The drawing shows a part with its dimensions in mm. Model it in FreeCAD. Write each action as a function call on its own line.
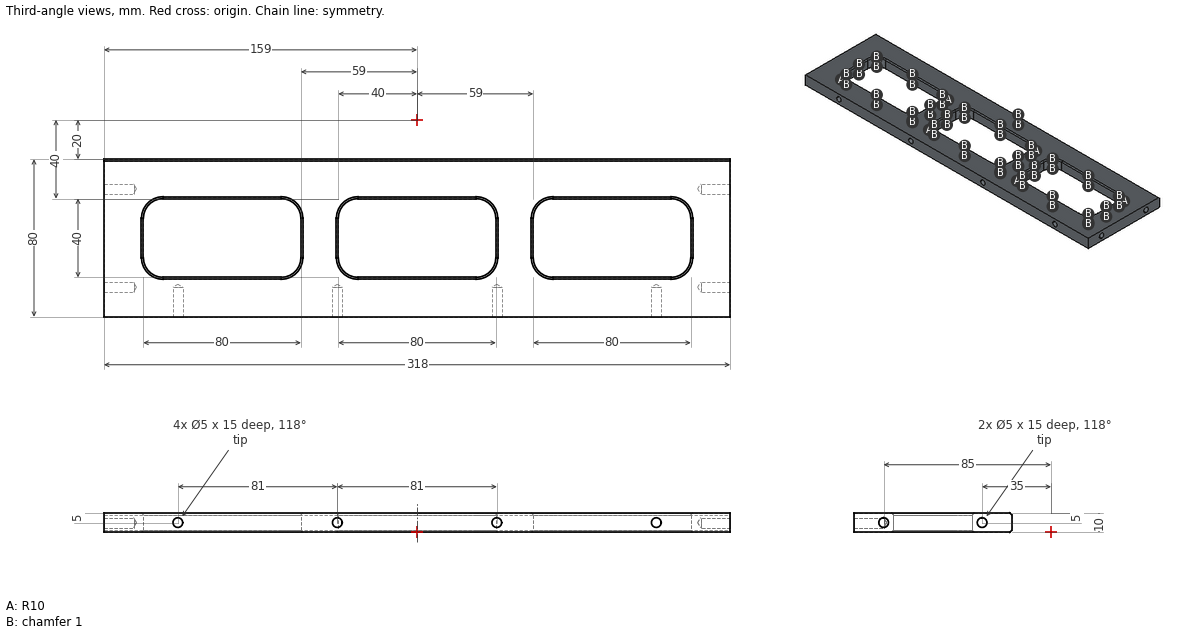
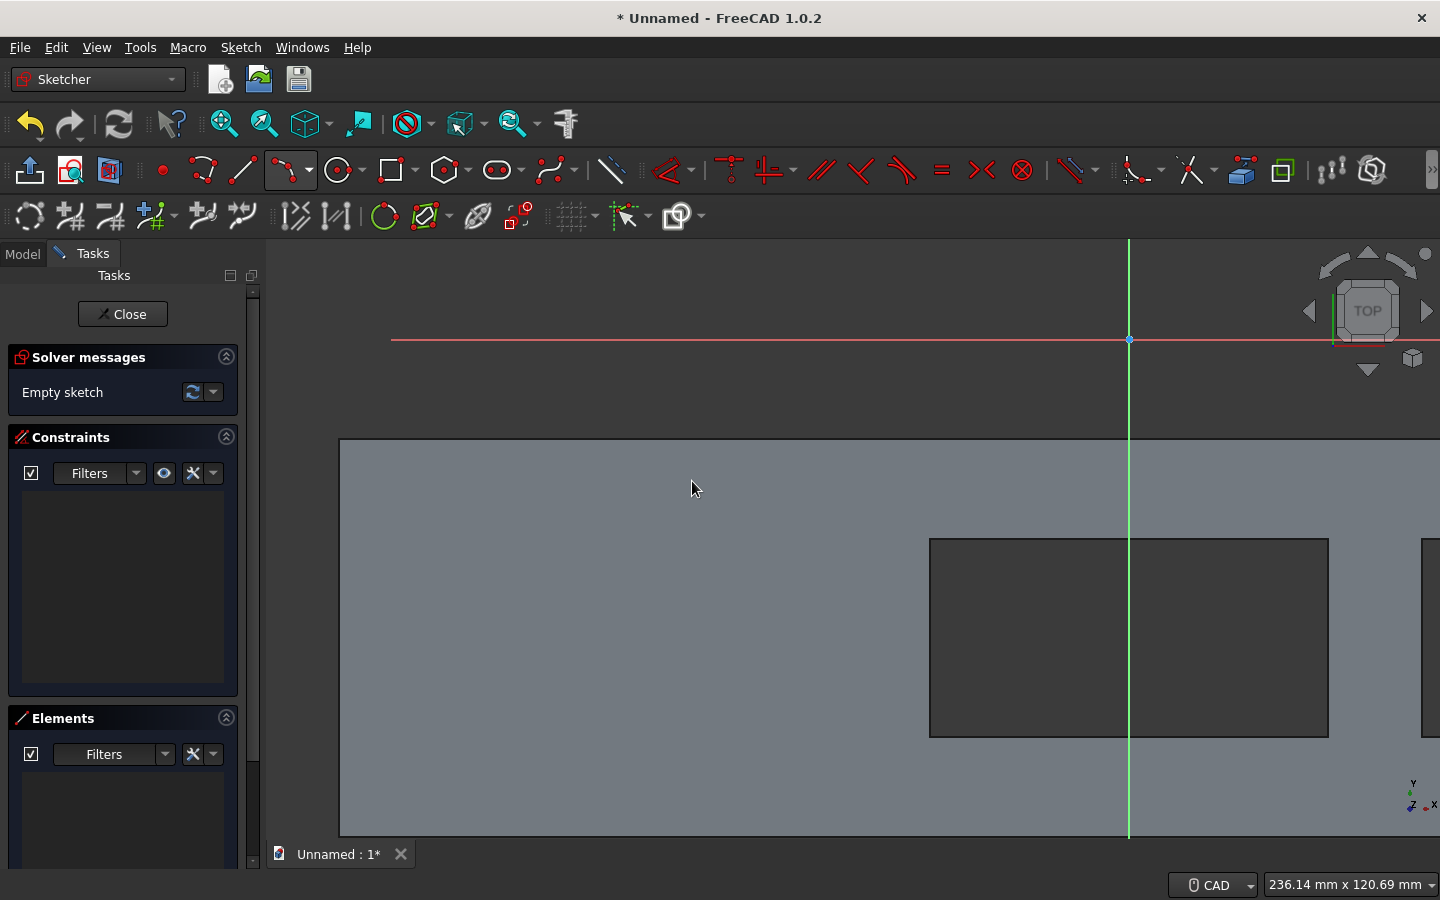
click(392, 170)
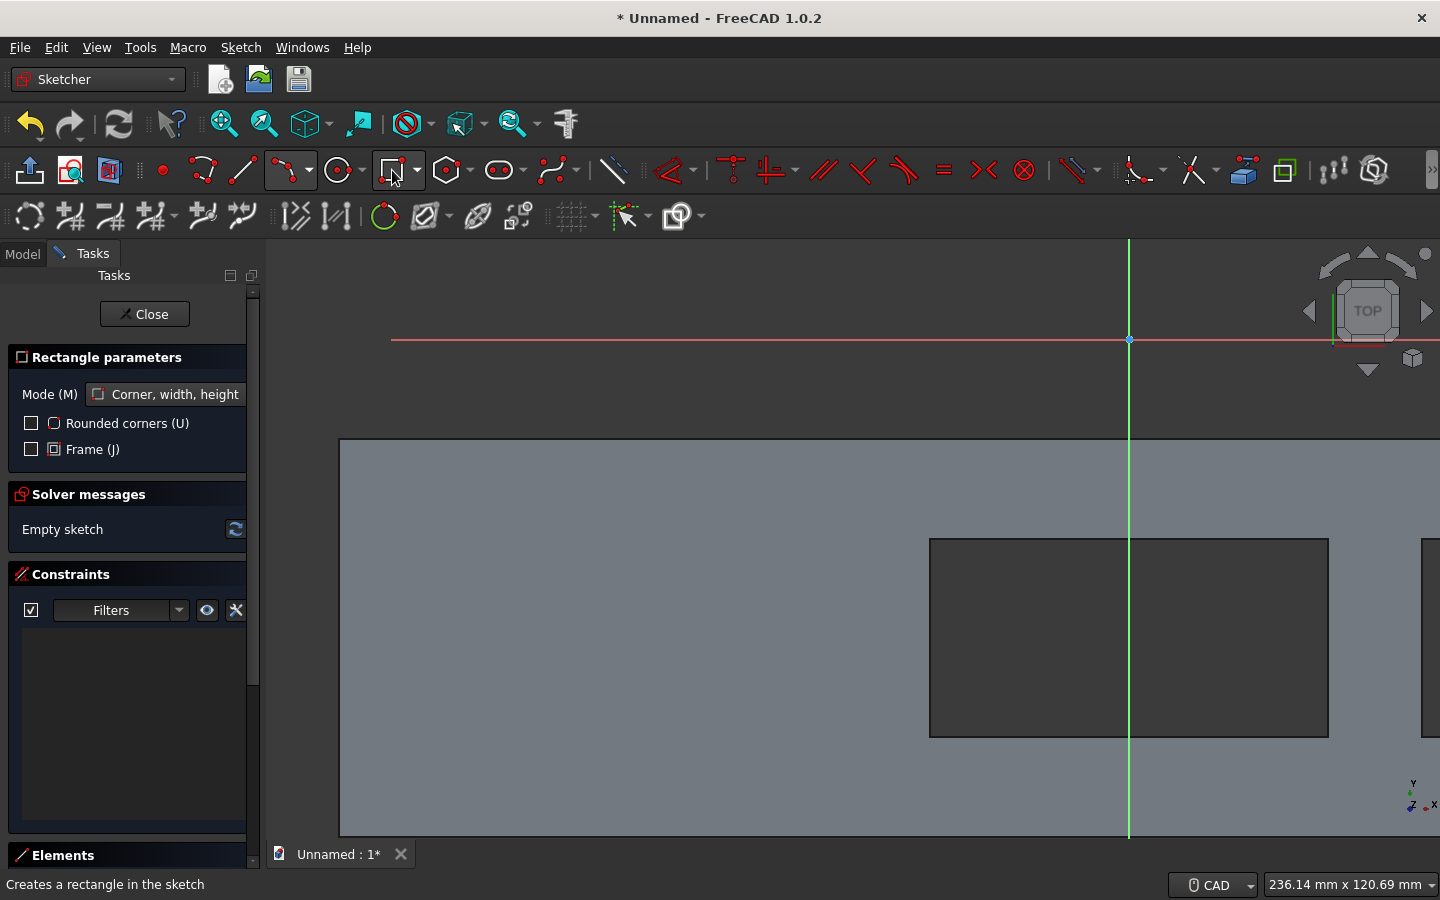
click(438, 539)
click(836, 737)
key(Escape)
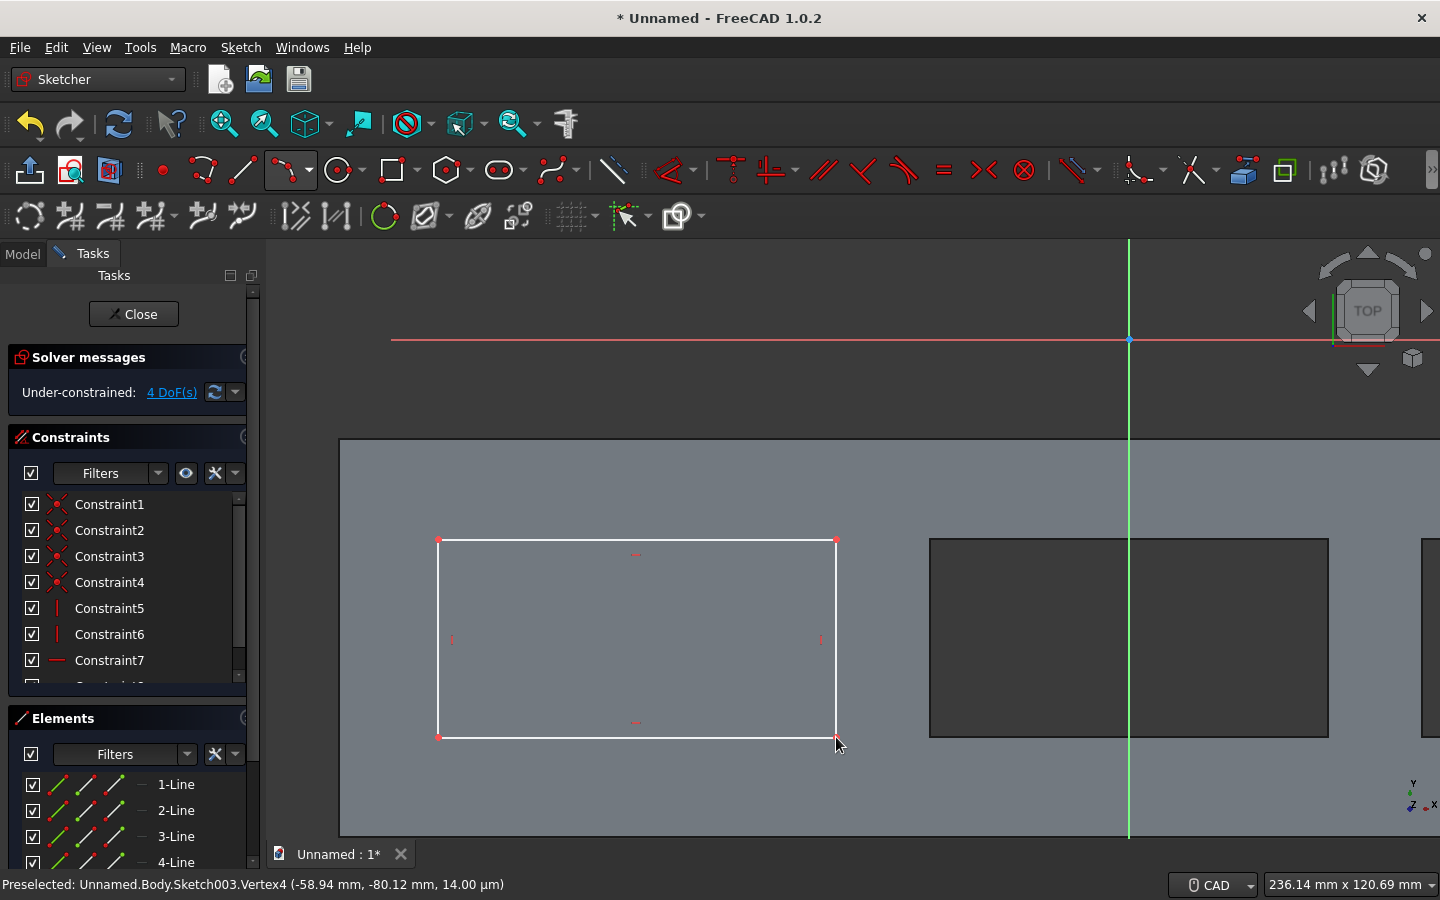
click(668, 170)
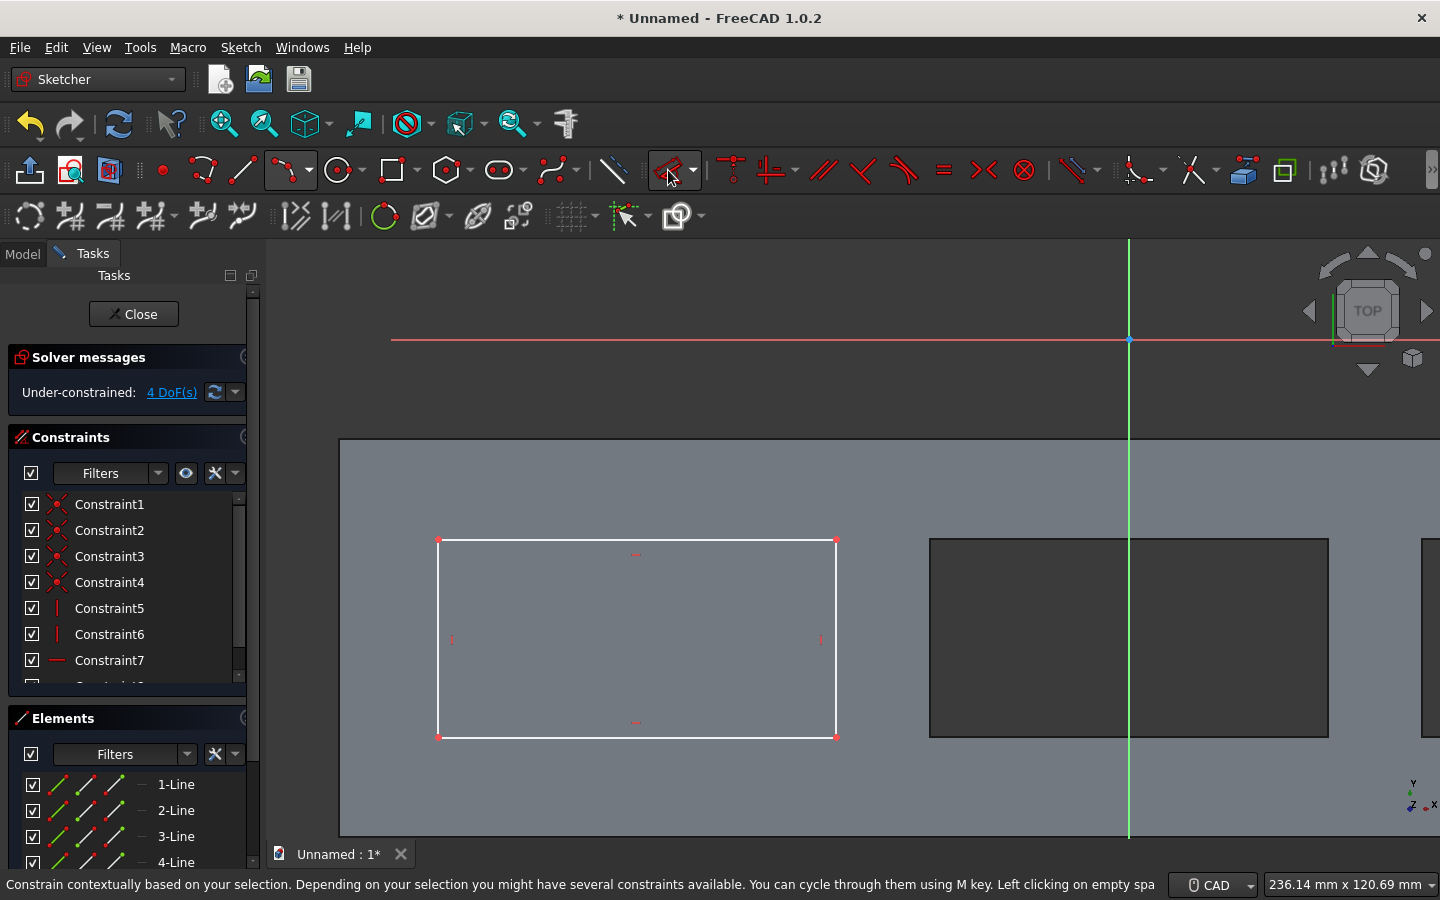
click(438, 599)
click(404, 639)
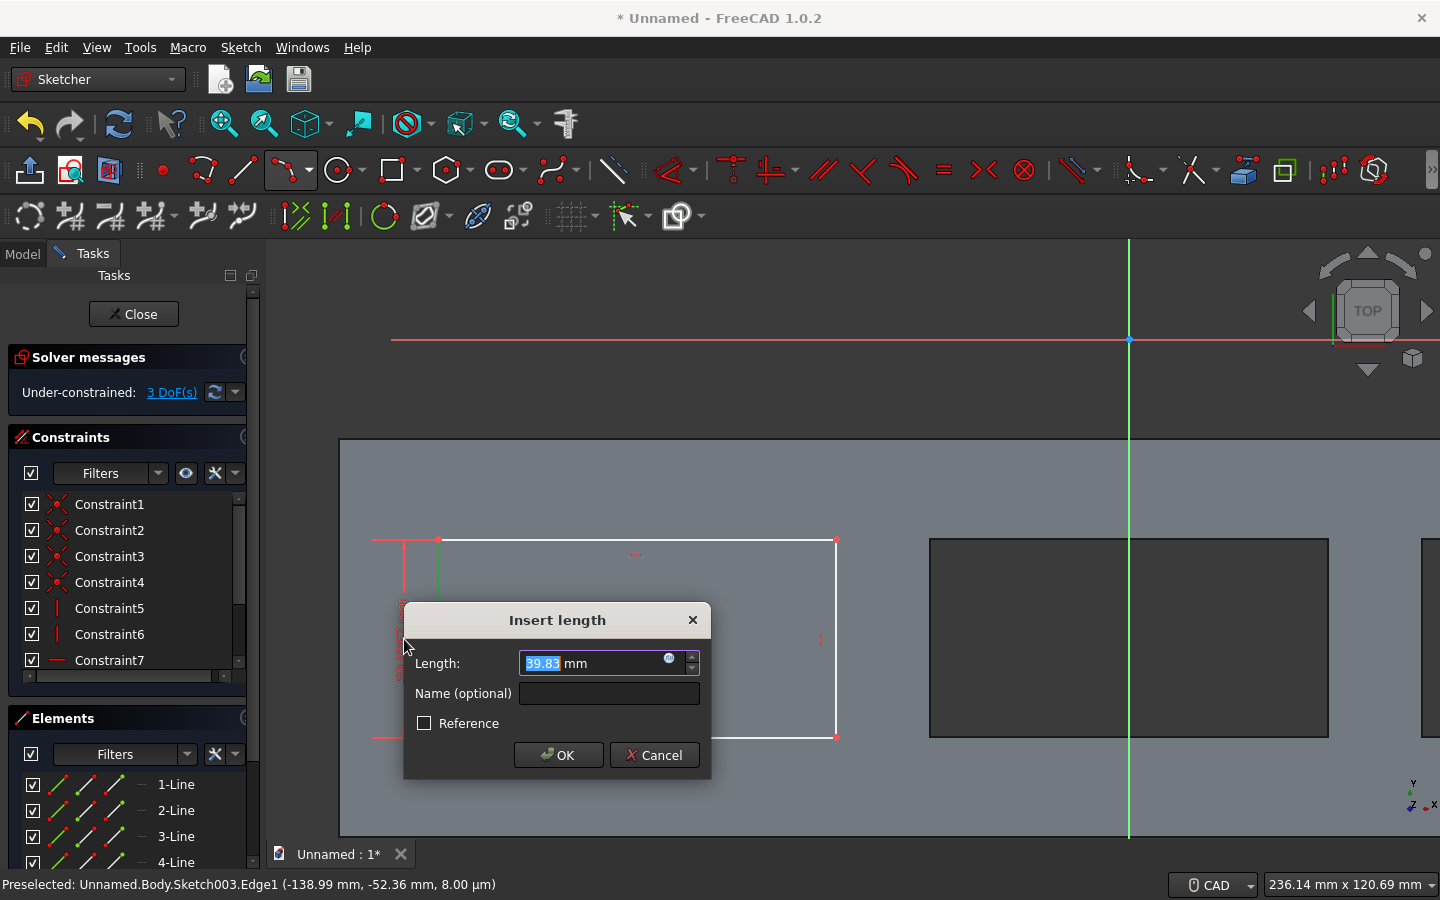
text(40)
key(Return)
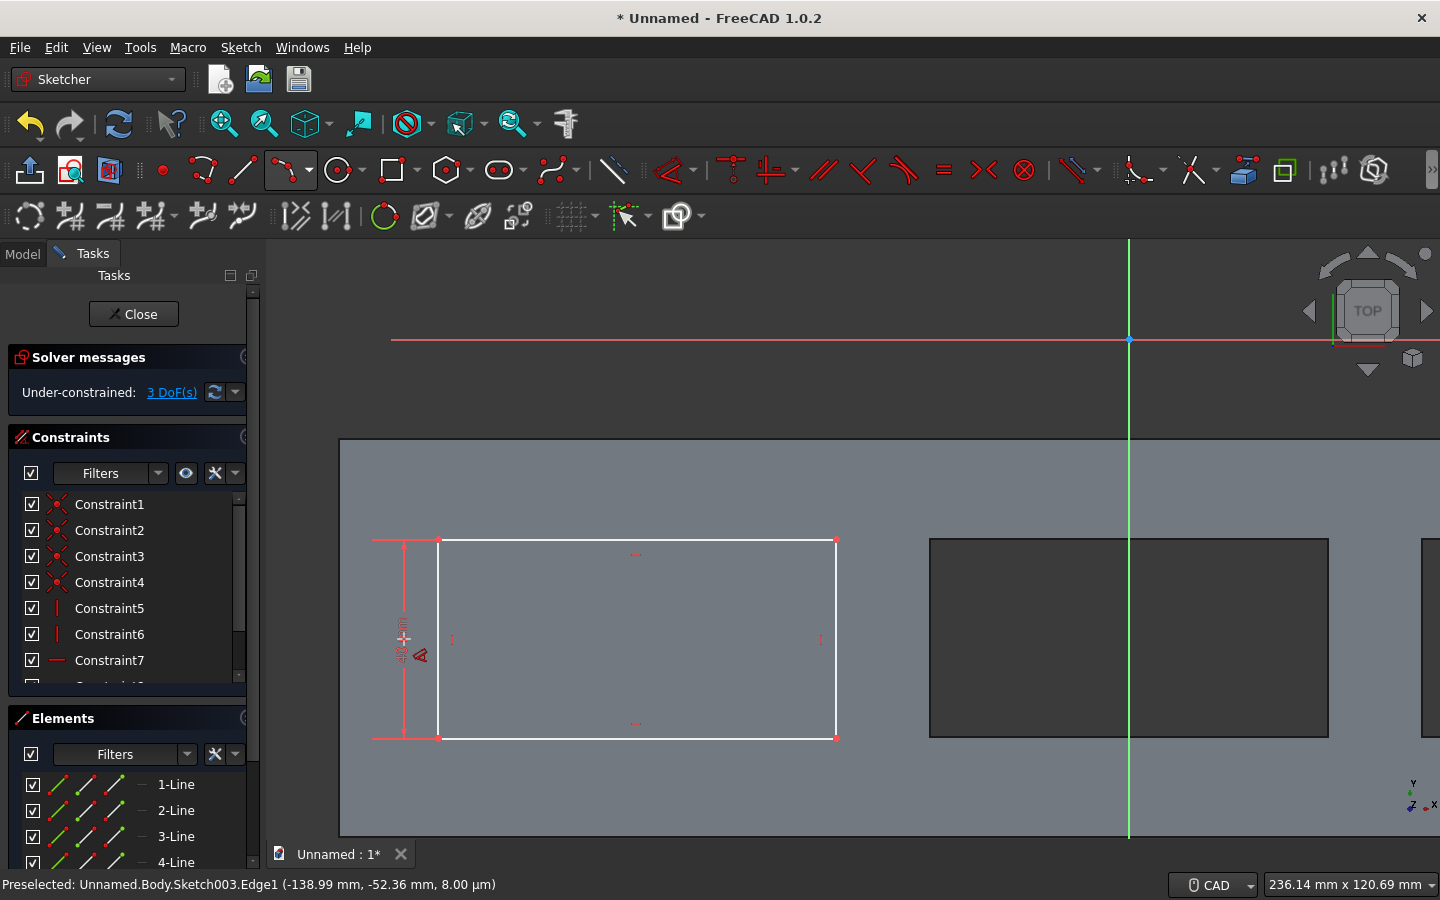
click(557, 739)
click(637, 773)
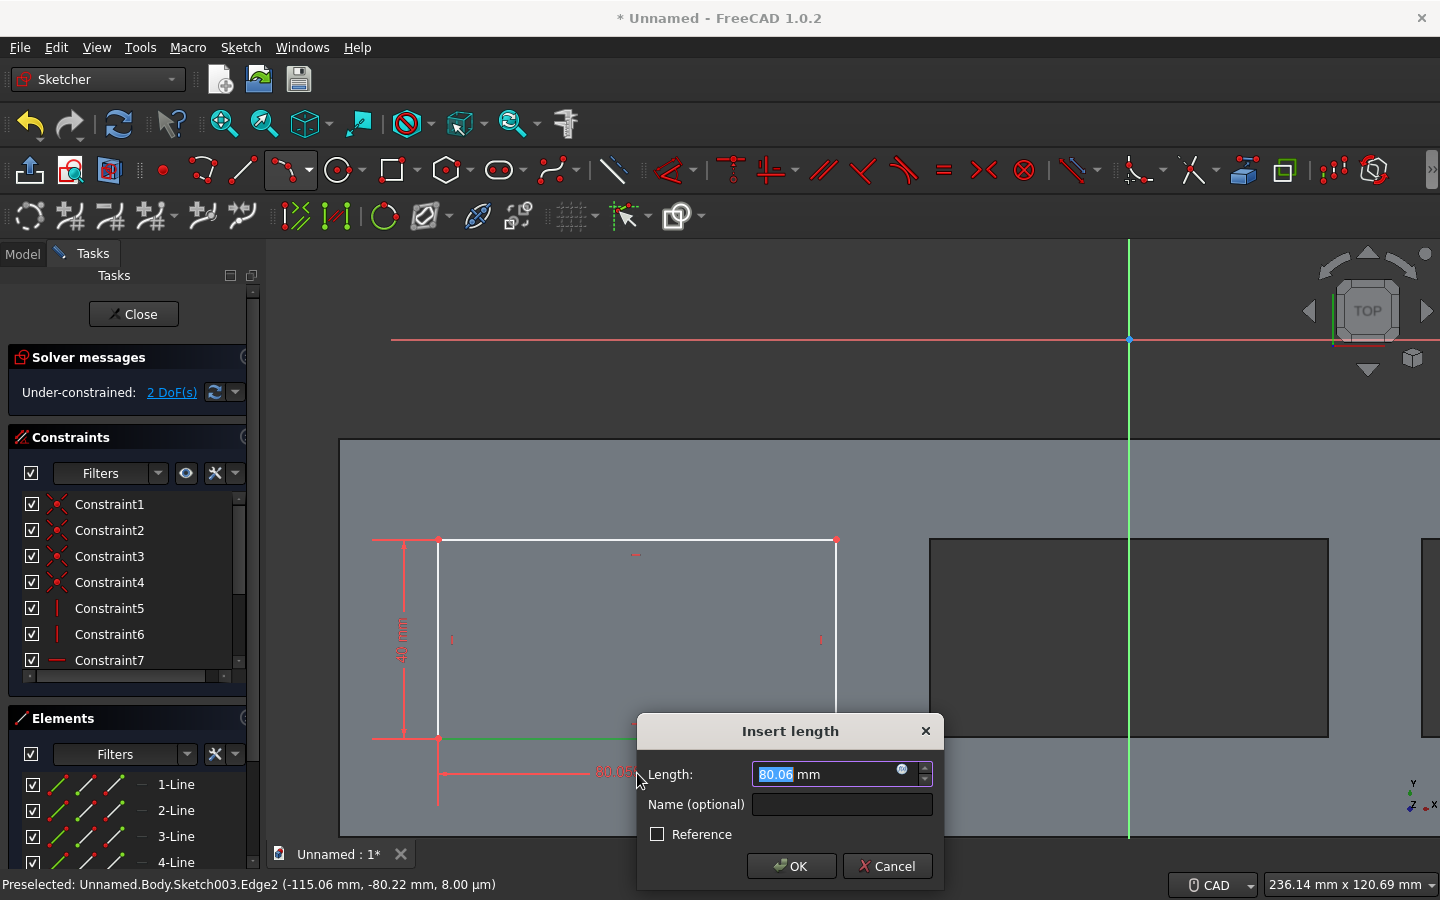
text(80)
key(Return)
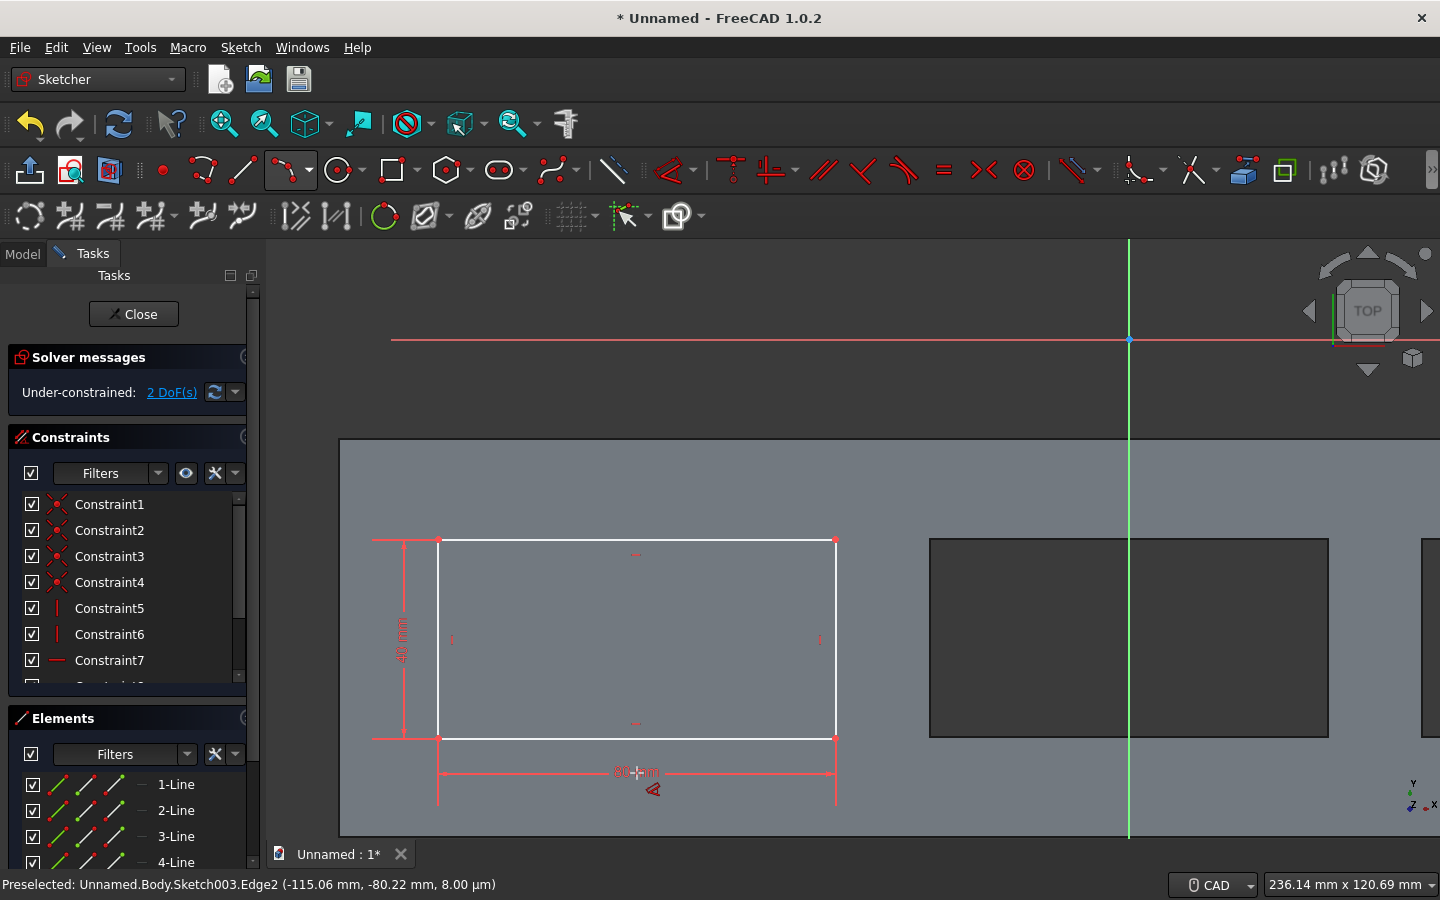
click(438, 540)
click(1163, 440)